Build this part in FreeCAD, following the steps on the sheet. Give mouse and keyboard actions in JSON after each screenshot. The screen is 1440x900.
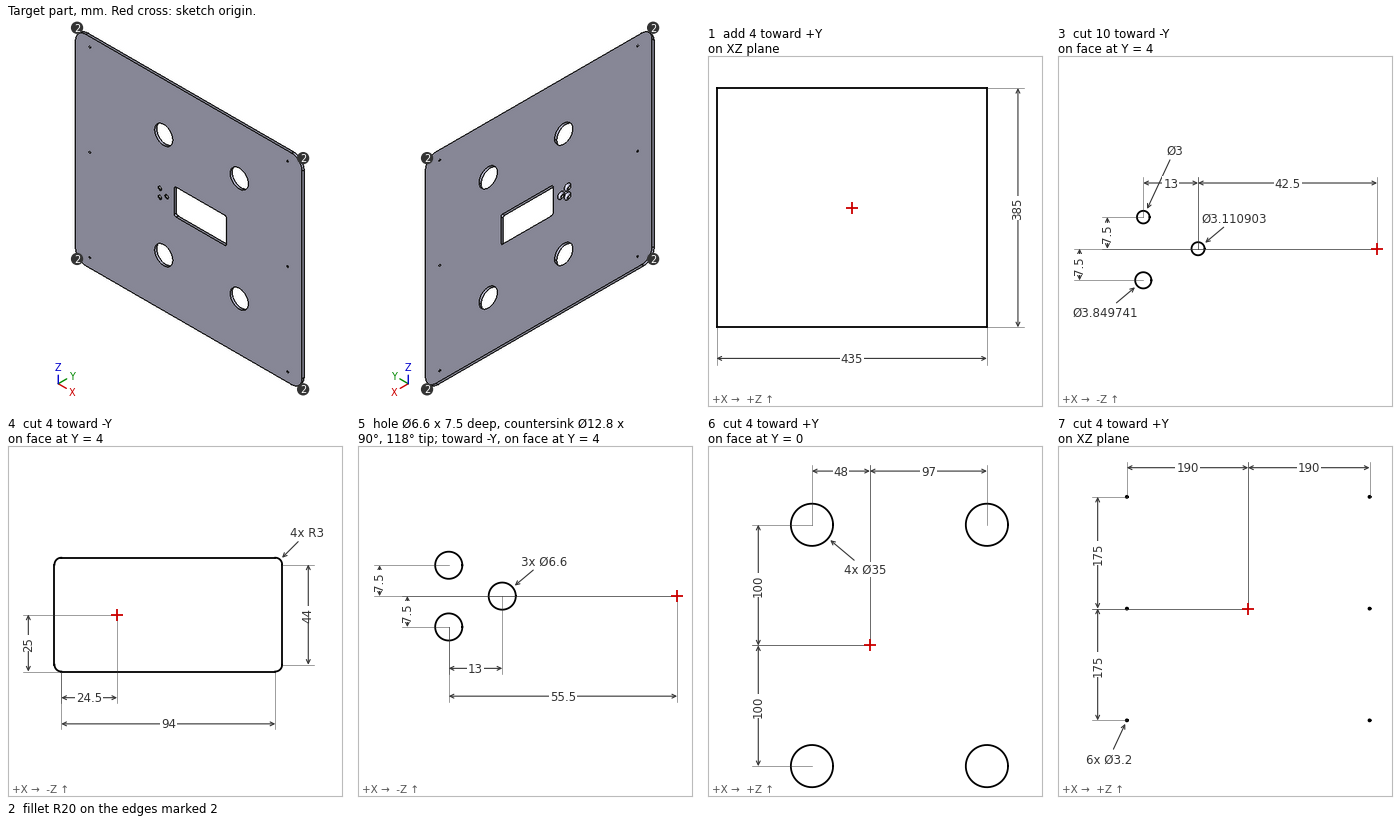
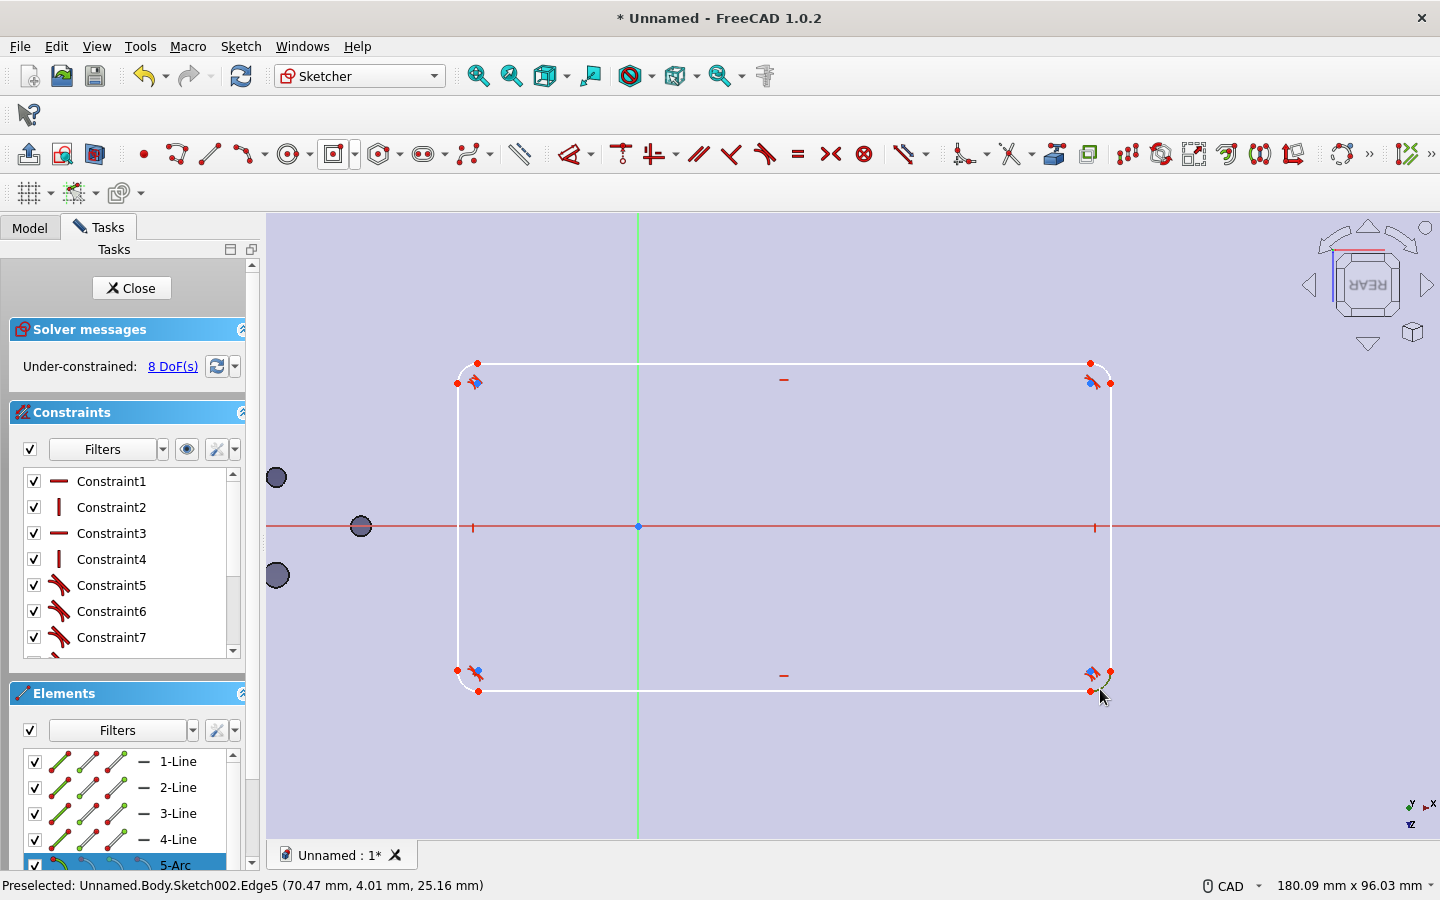
{"action": "scroll", "coordinate": [1109, 375], "scroll_direction": "up", "scroll_amount": 2}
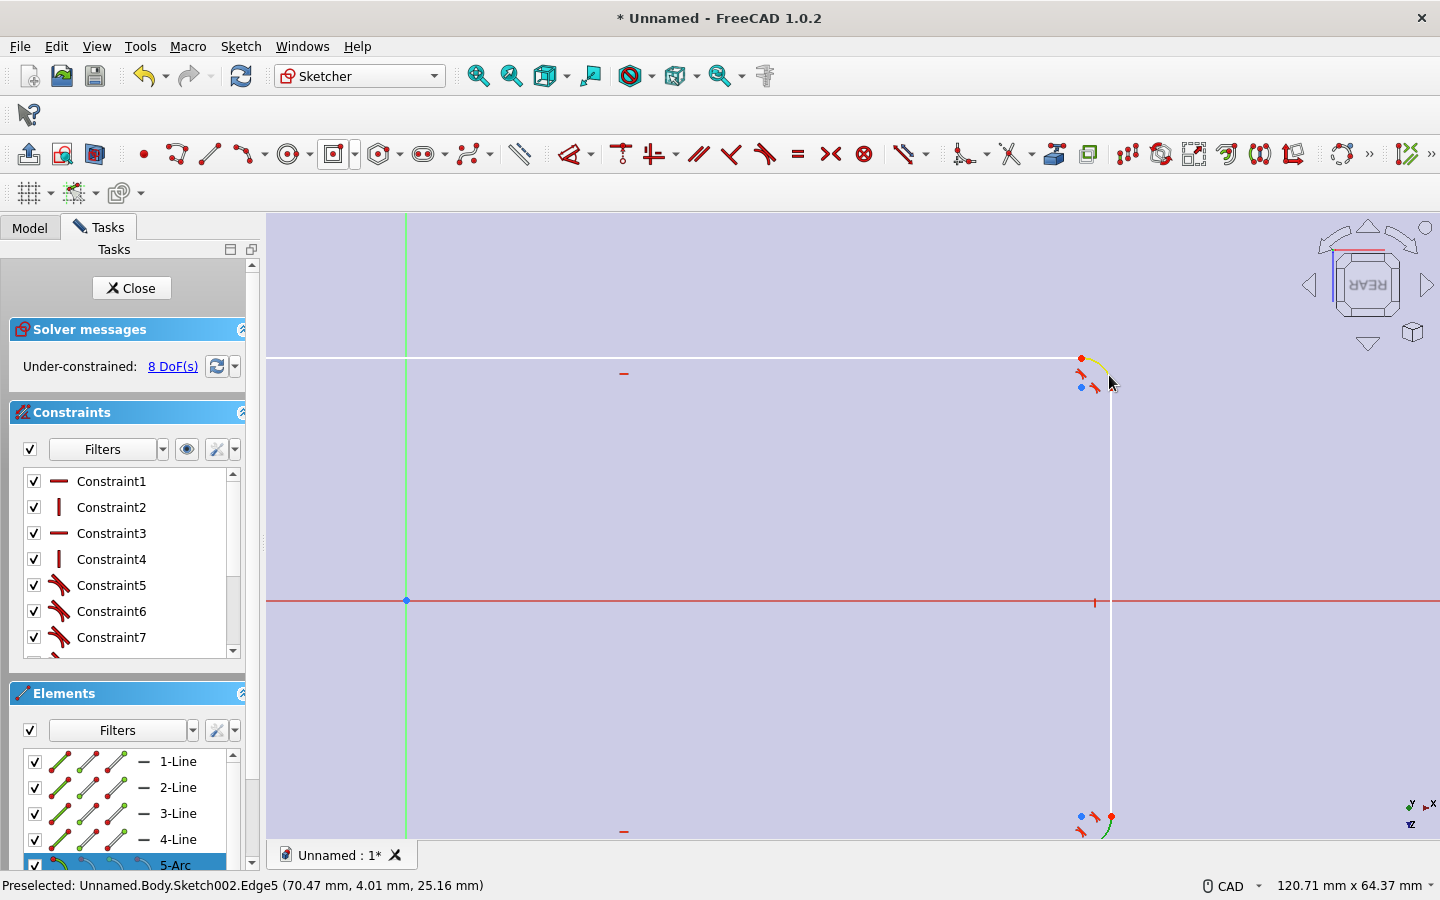
{"action": "left_click", "coordinate": [1108, 374]}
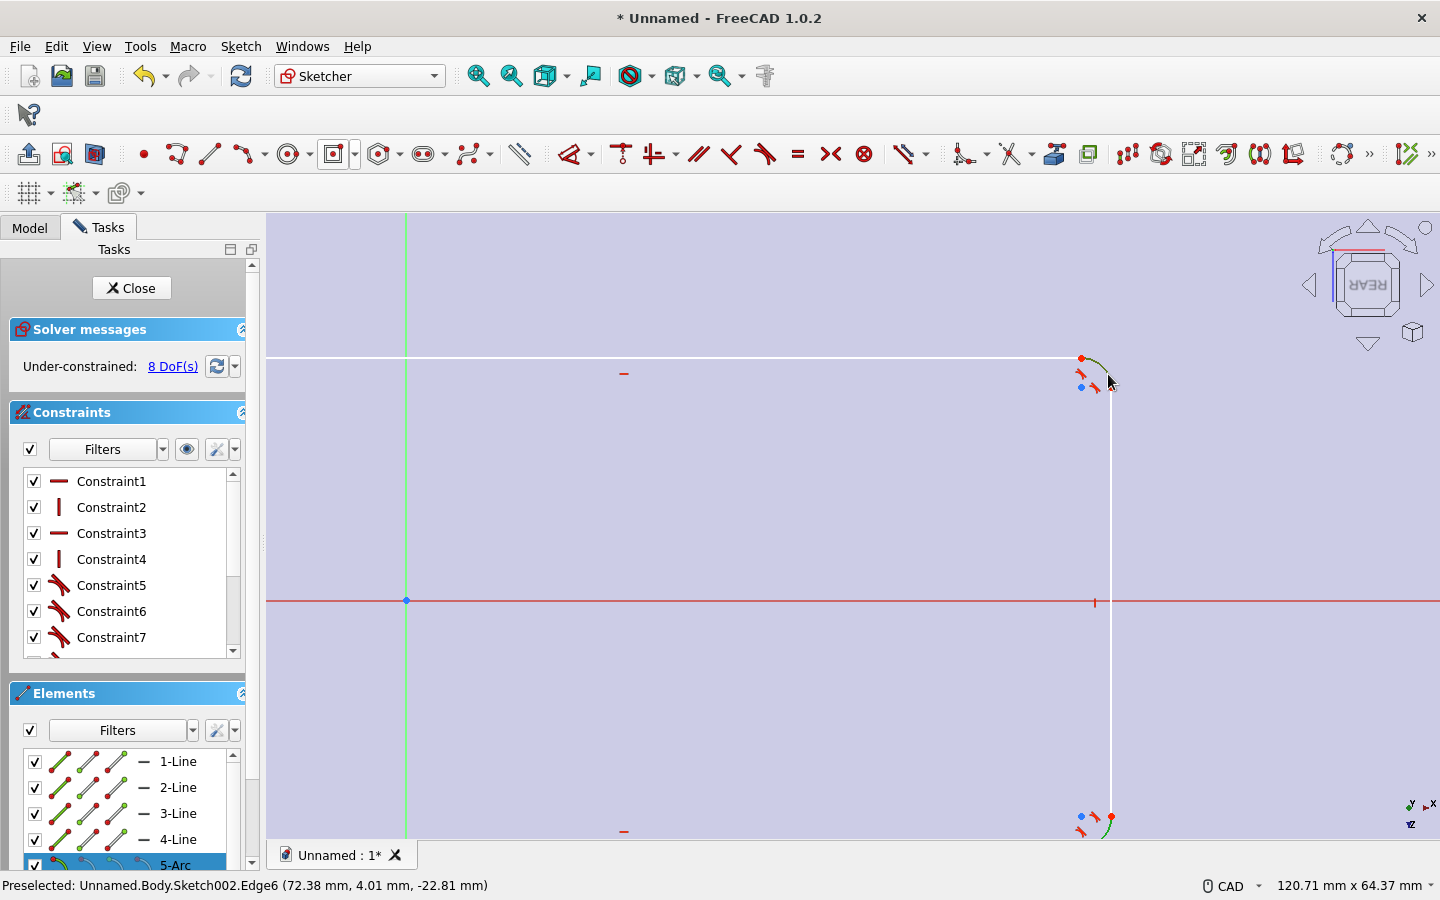
{"action": "scroll", "coordinate": [1109, 374], "scroll_direction": "down", "scroll_amount": 2}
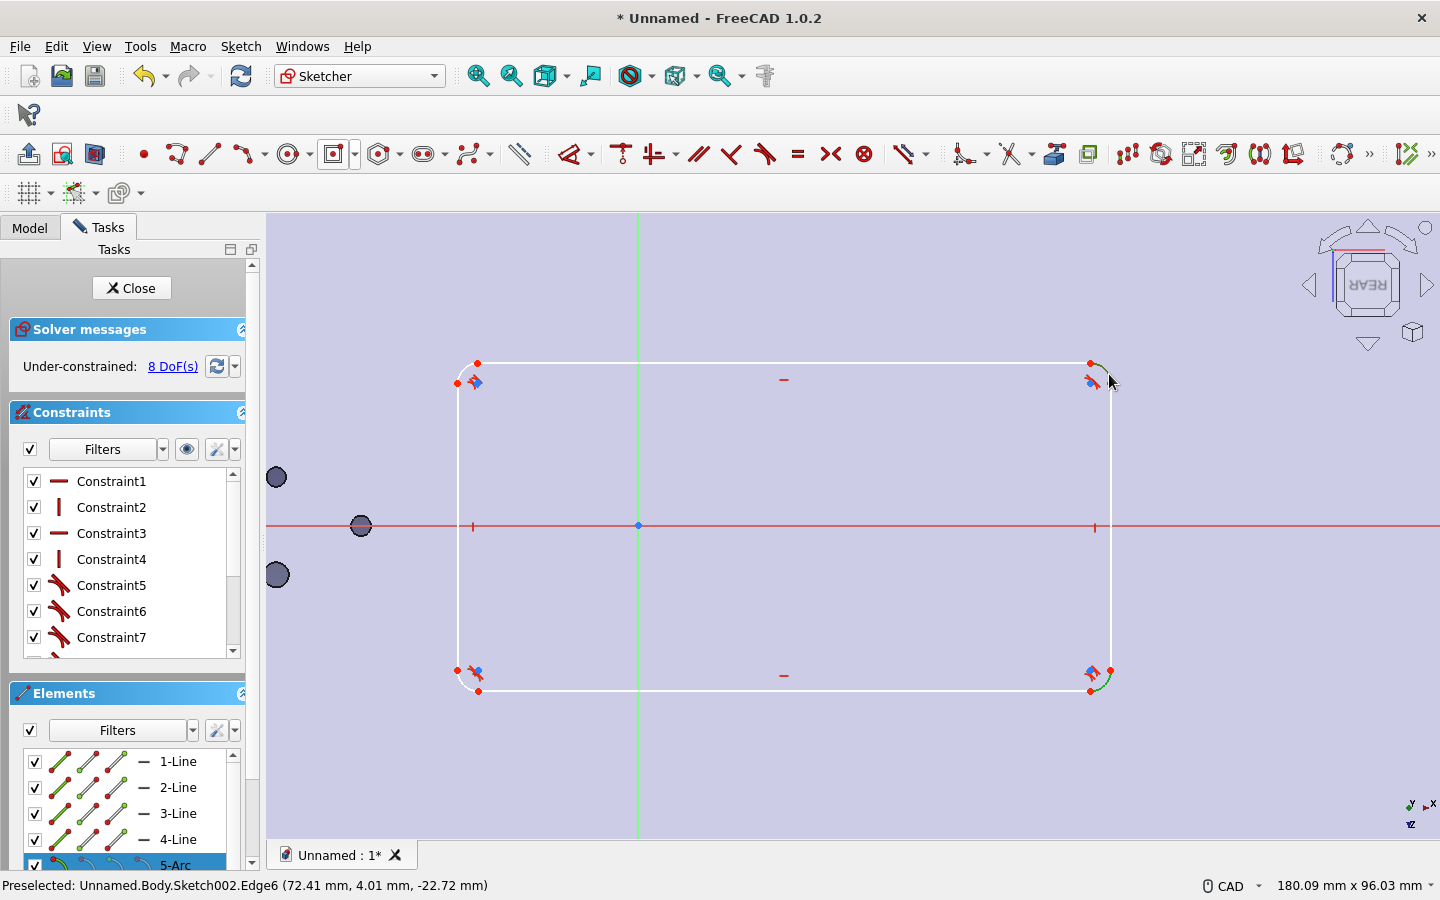
{"action": "scroll", "coordinate": [469, 366], "scroll_direction": "up", "scroll_amount": 2}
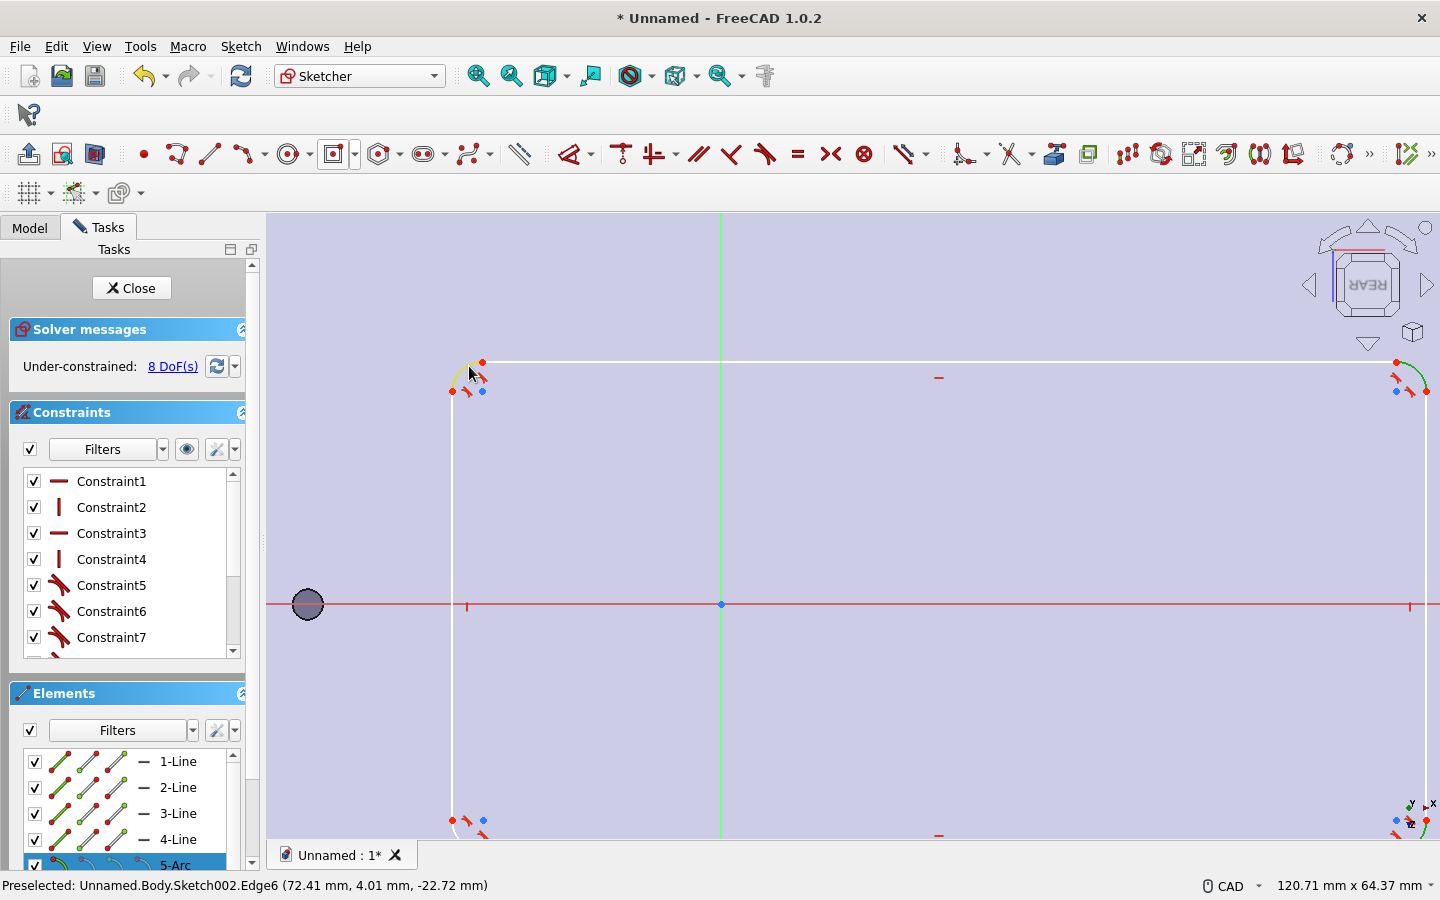
{"action": "left_click", "coordinate": [469, 365]}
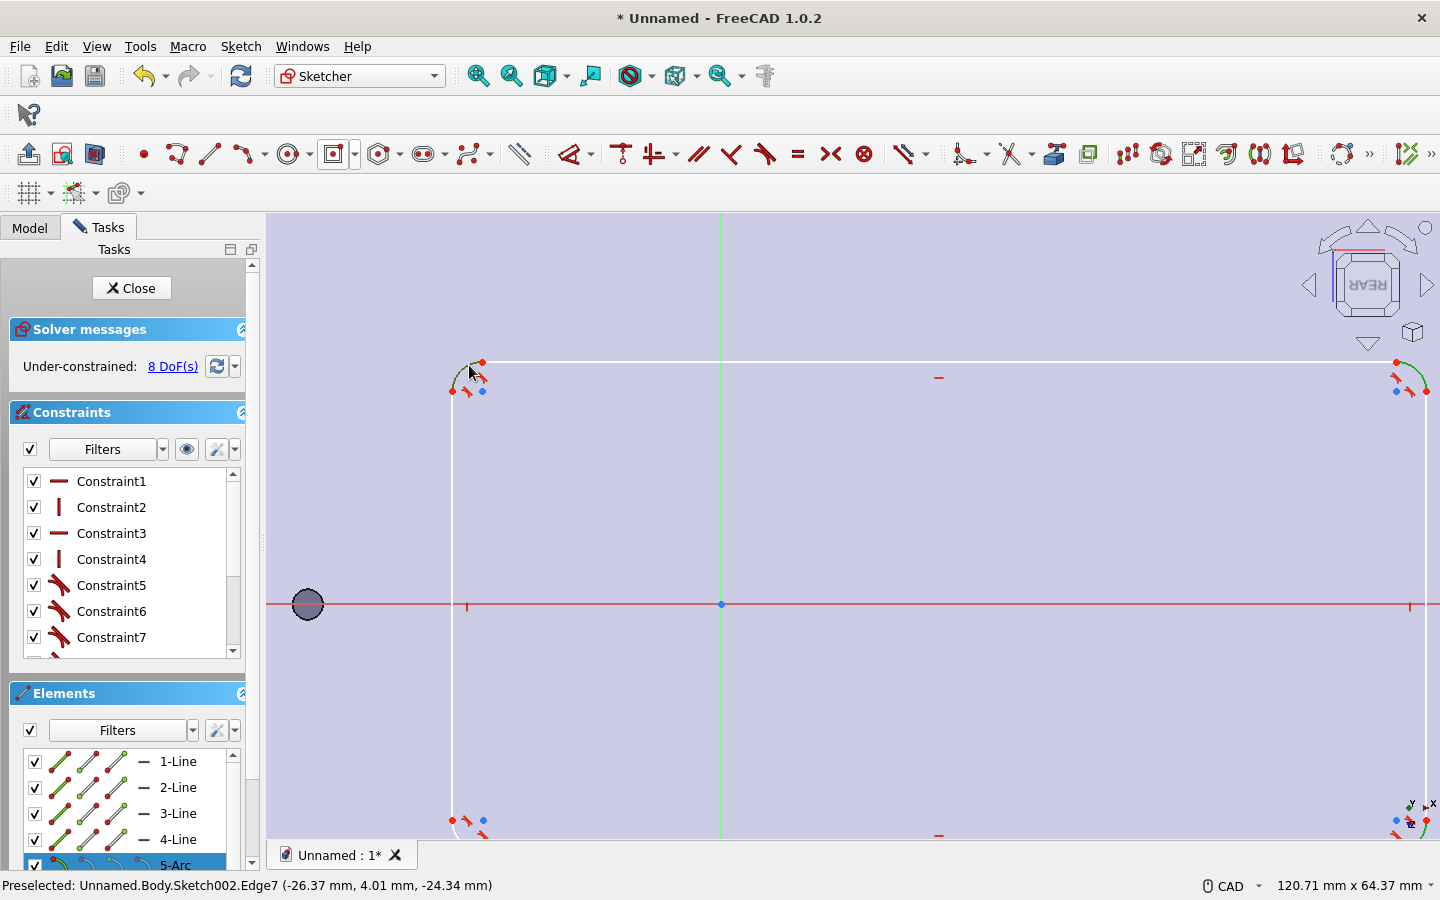
{"action": "scroll", "coordinate": [468, 366], "scroll_direction": "down", "scroll_amount": 2}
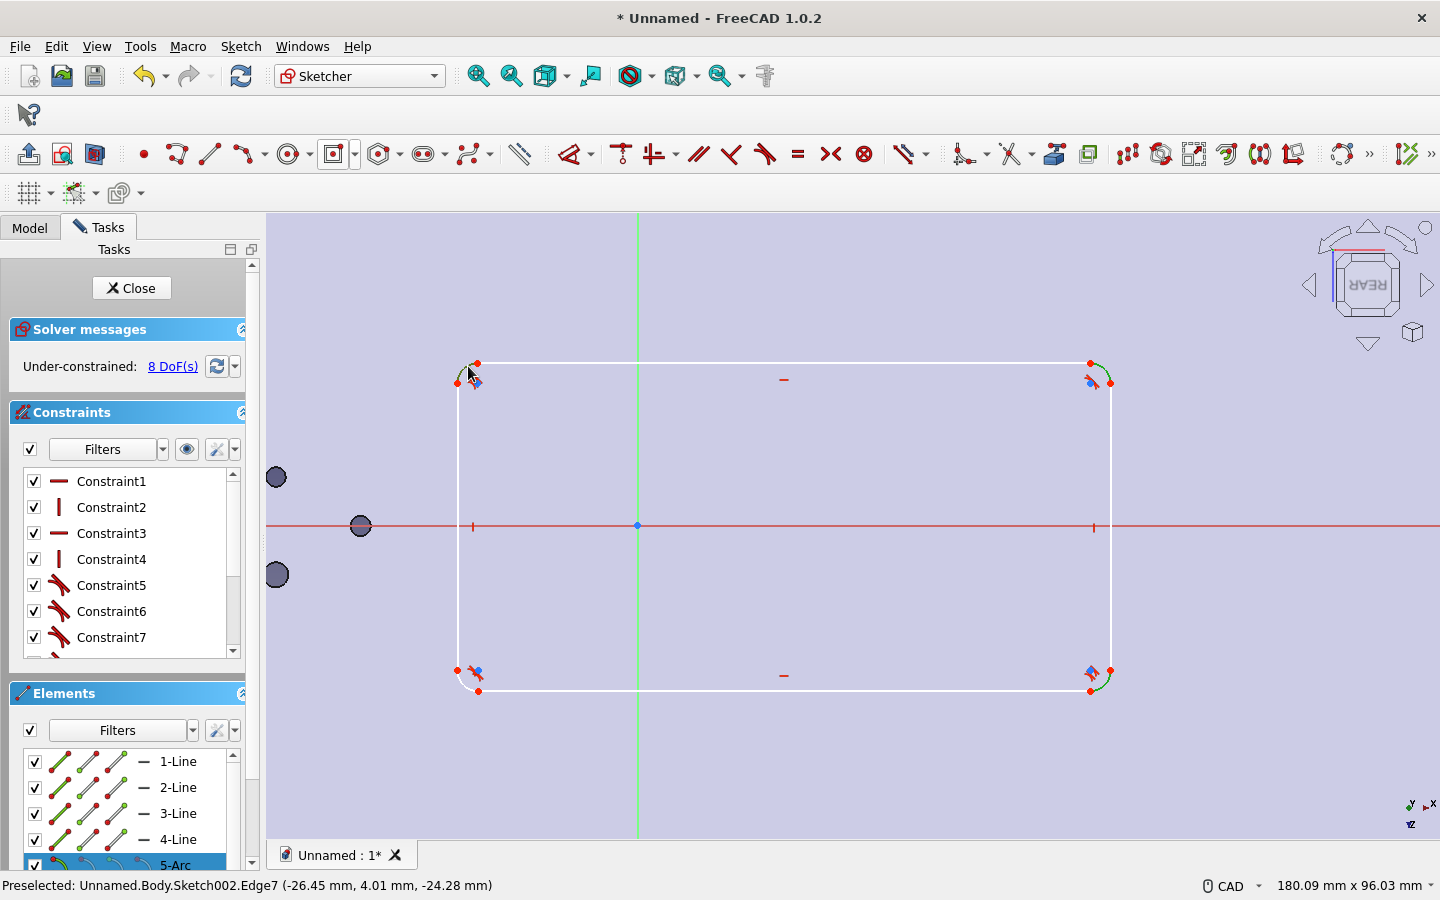
{"action": "scroll", "coordinate": [460, 680], "scroll_direction": "up", "scroll_amount": 2}